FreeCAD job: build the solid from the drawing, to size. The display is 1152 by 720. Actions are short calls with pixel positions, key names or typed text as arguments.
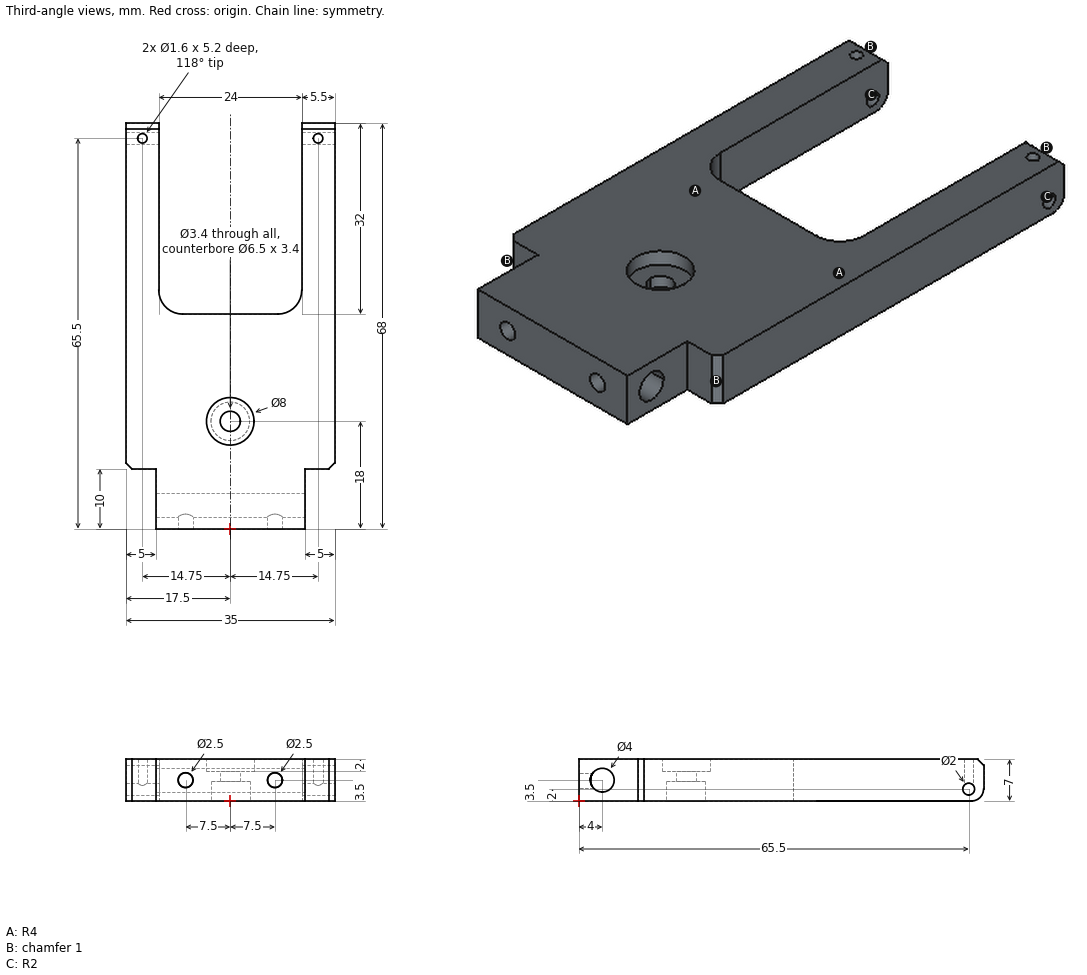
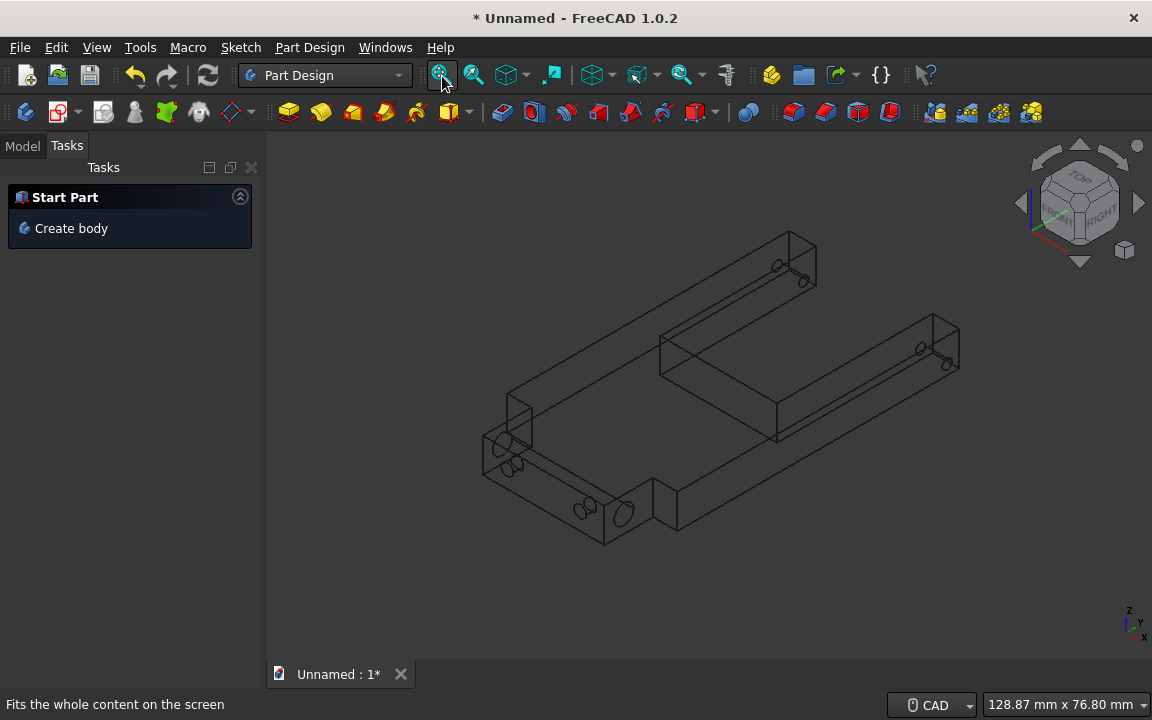
click(660, 355)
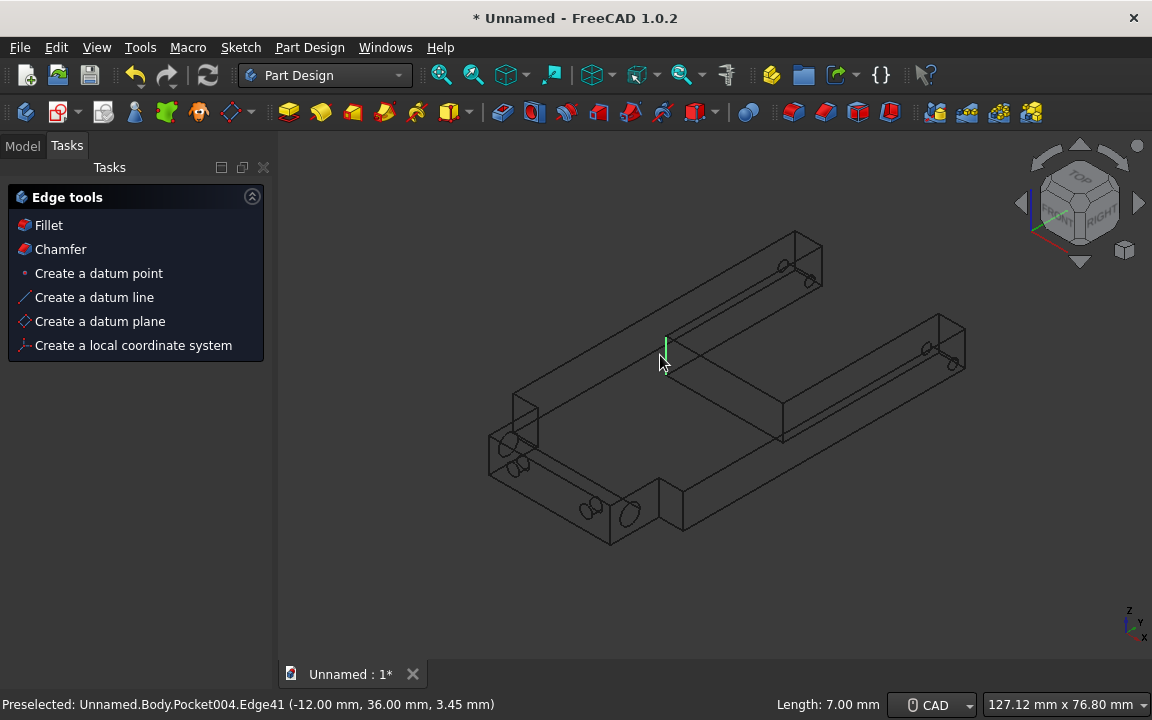
click(783, 422, ctrl)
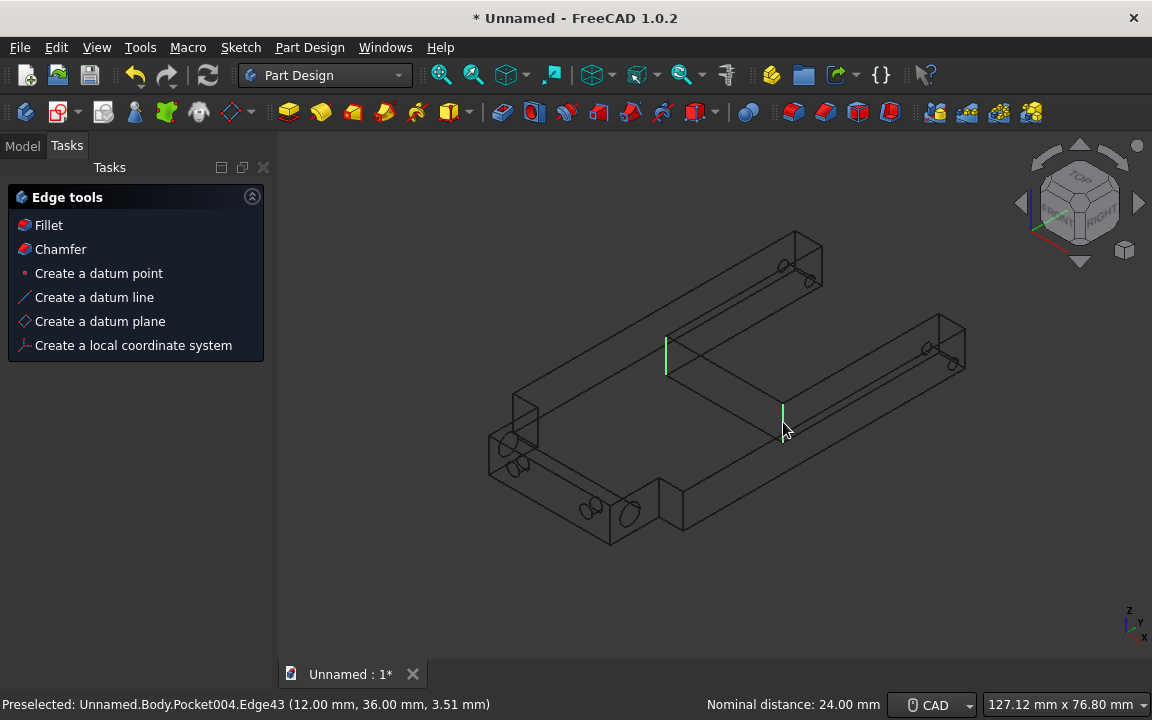
key(v)
key(1)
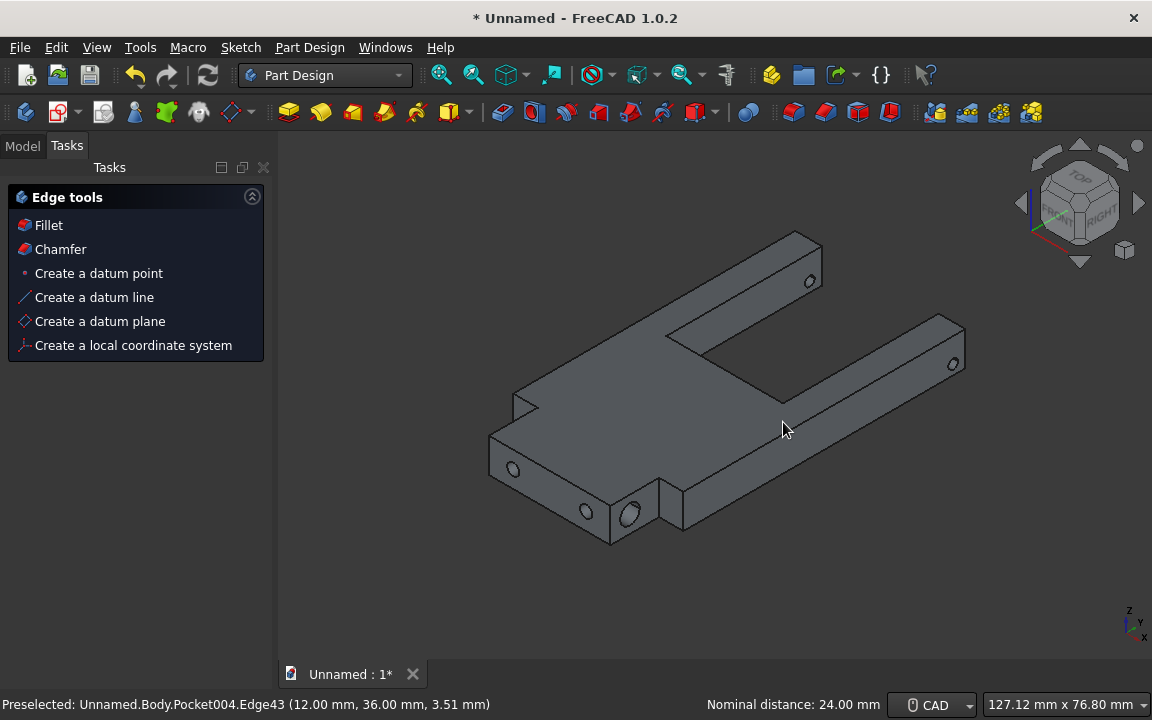
click(794, 112)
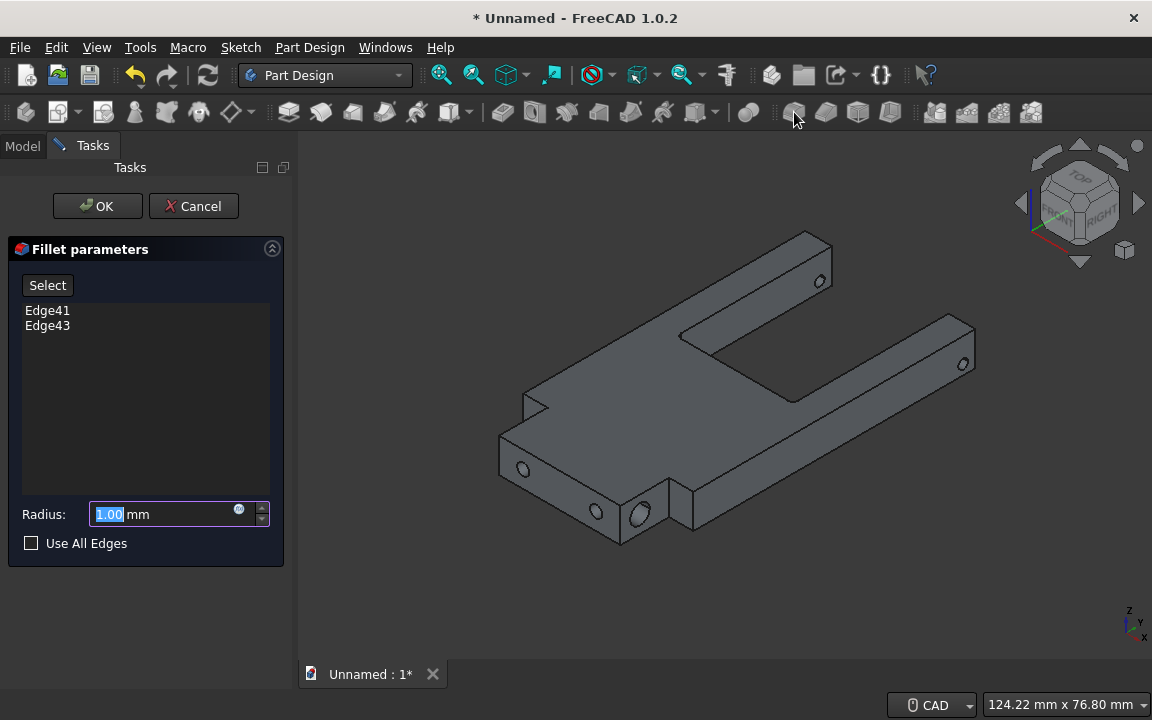
text(4)
key(Tab)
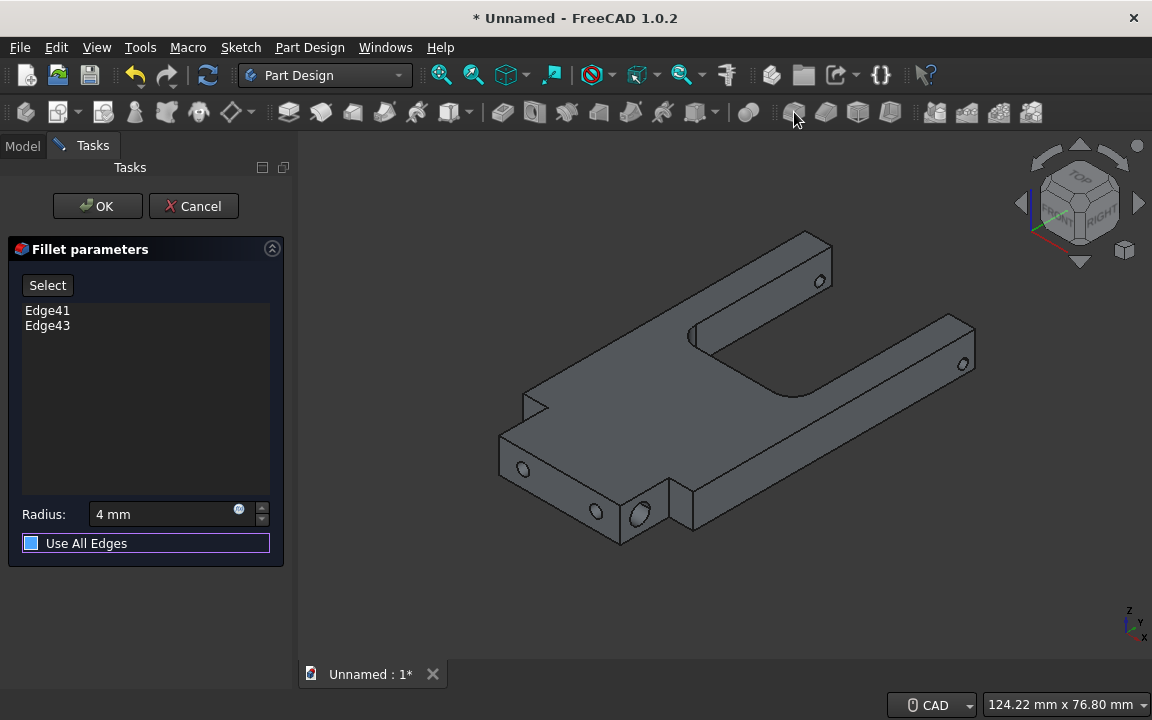
click(98, 206)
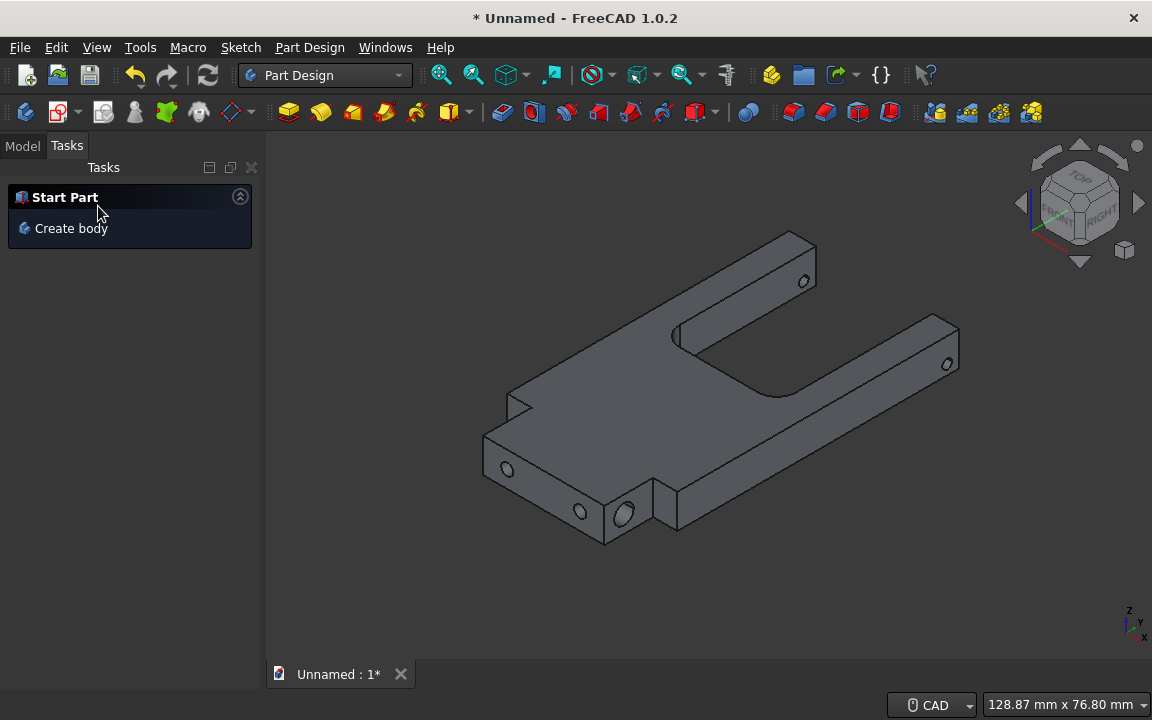
click(677, 510)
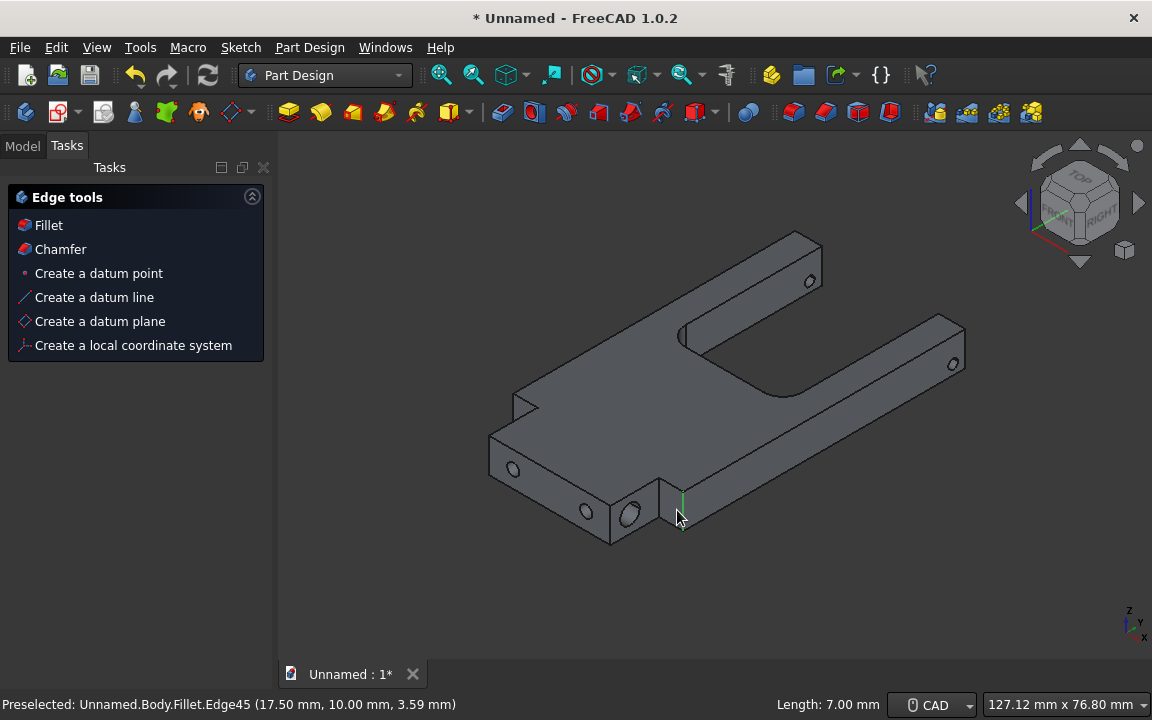
key(2)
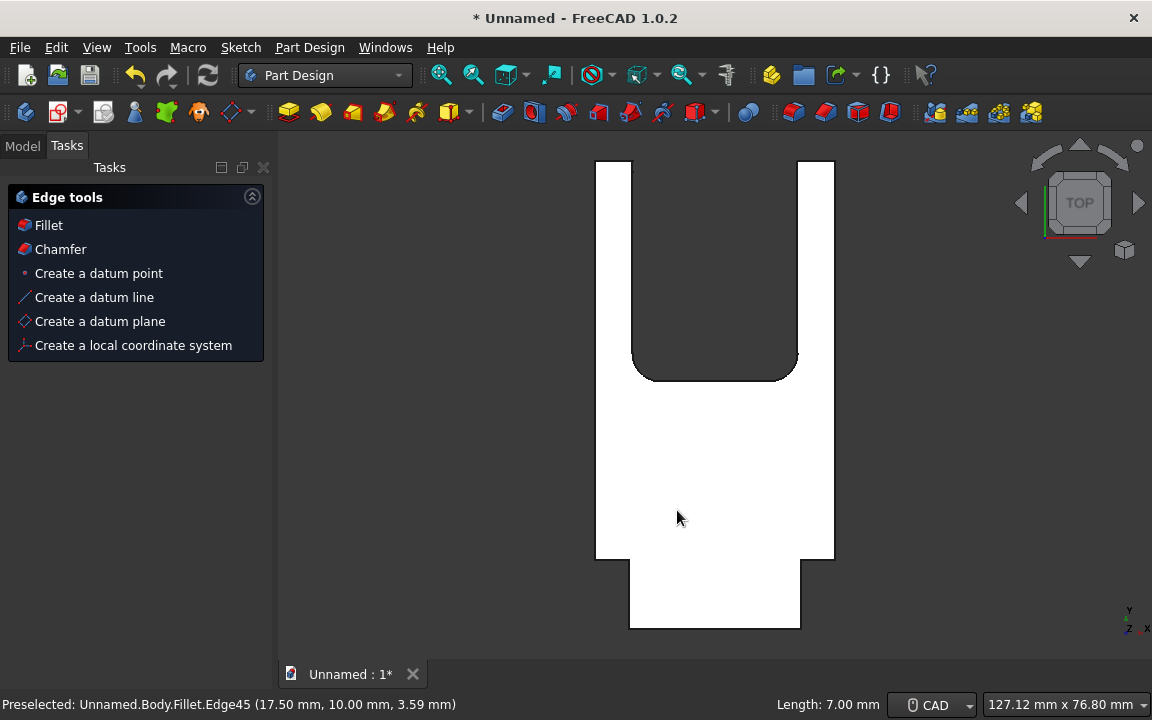
click(816, 160, ctrl)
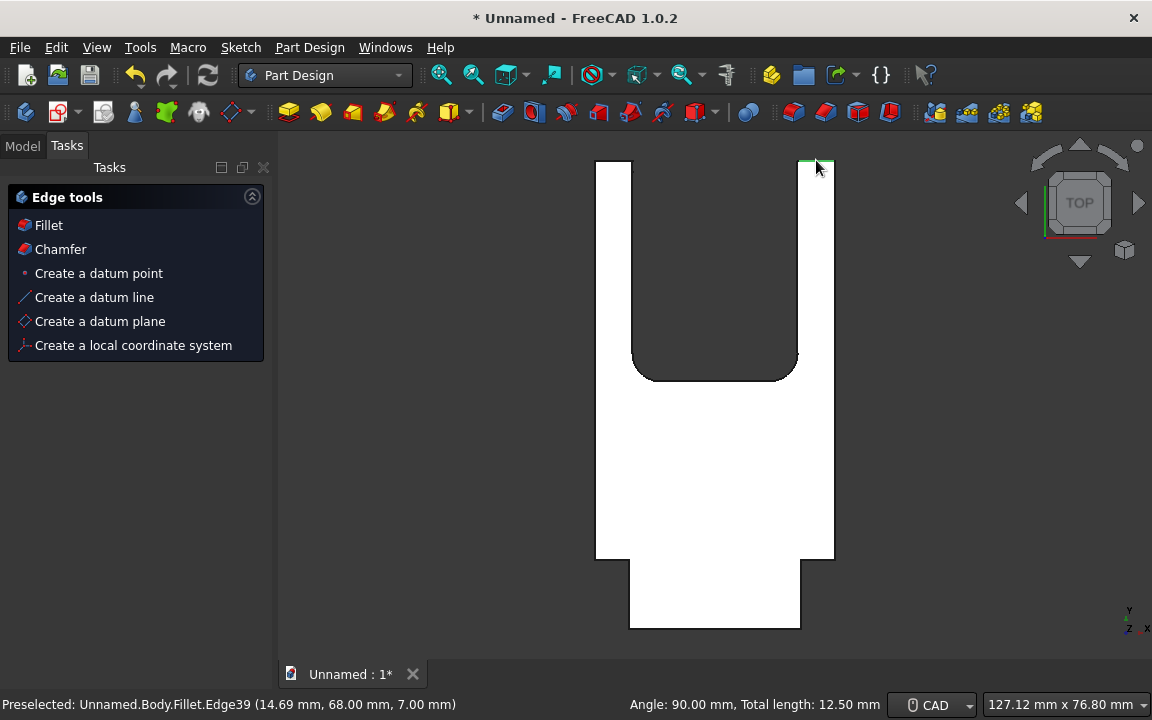
click(614, 160, ctrl)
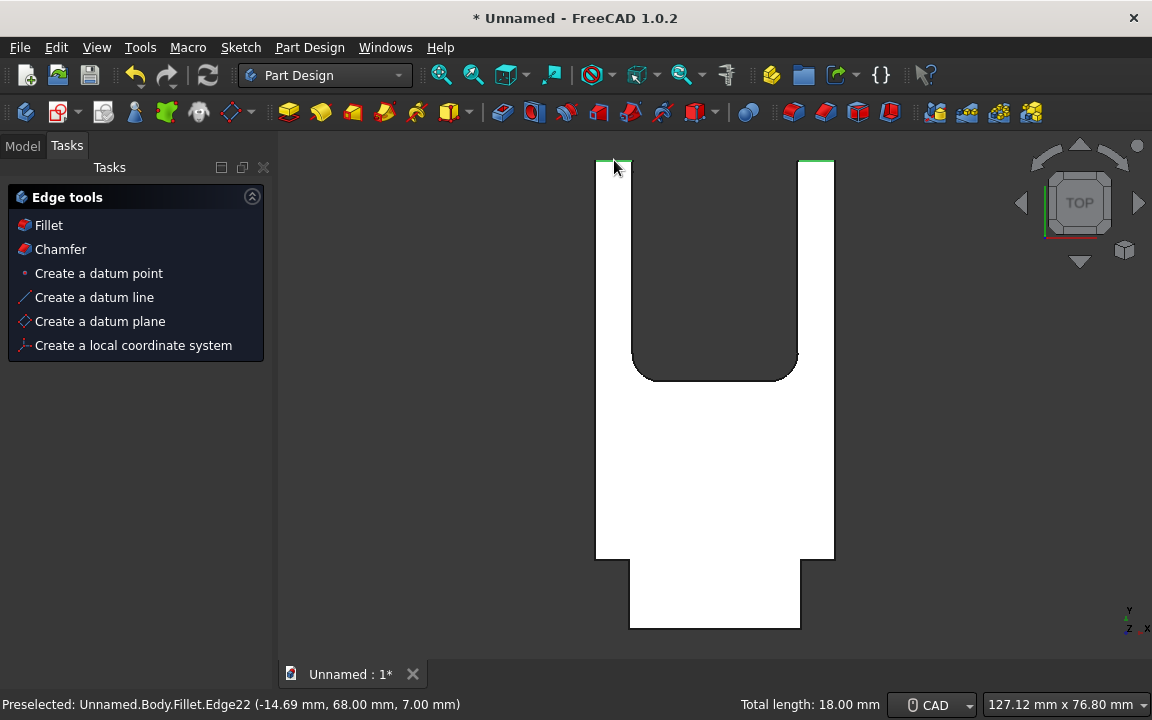
key(0)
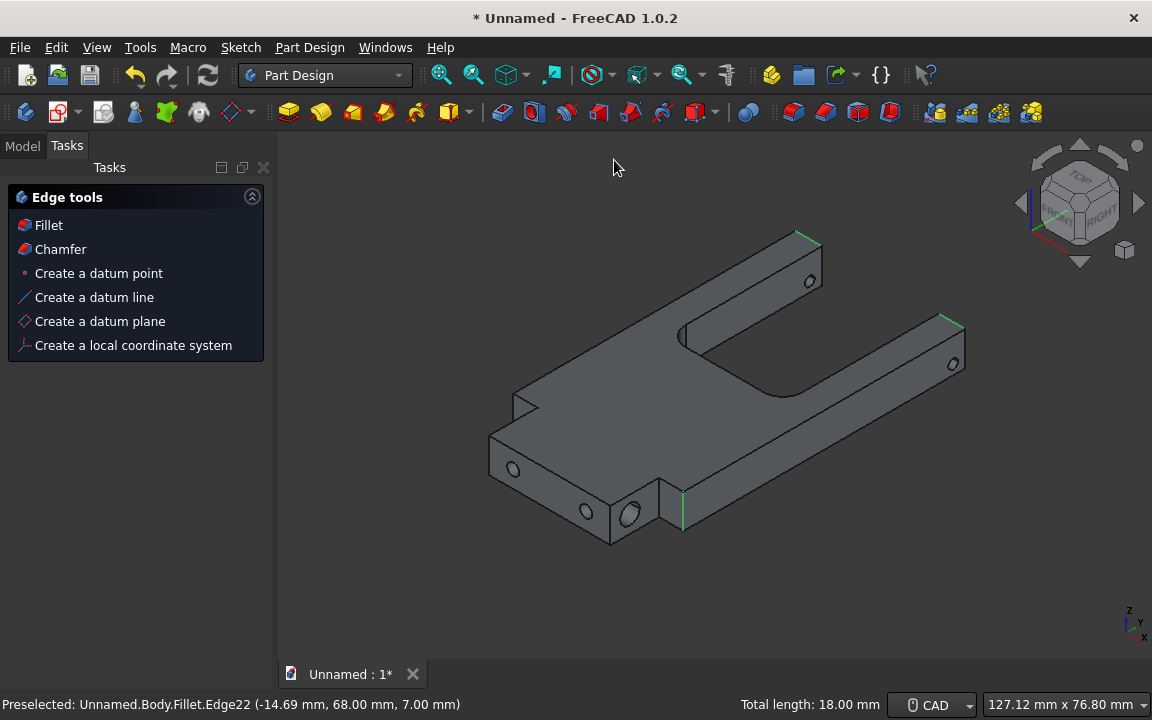
key(1)